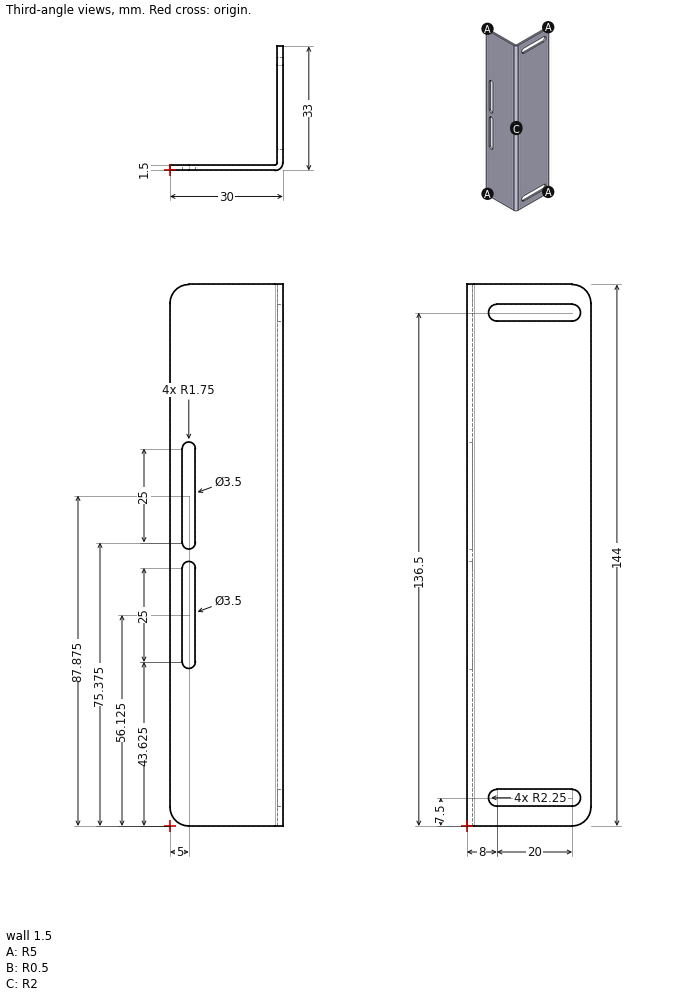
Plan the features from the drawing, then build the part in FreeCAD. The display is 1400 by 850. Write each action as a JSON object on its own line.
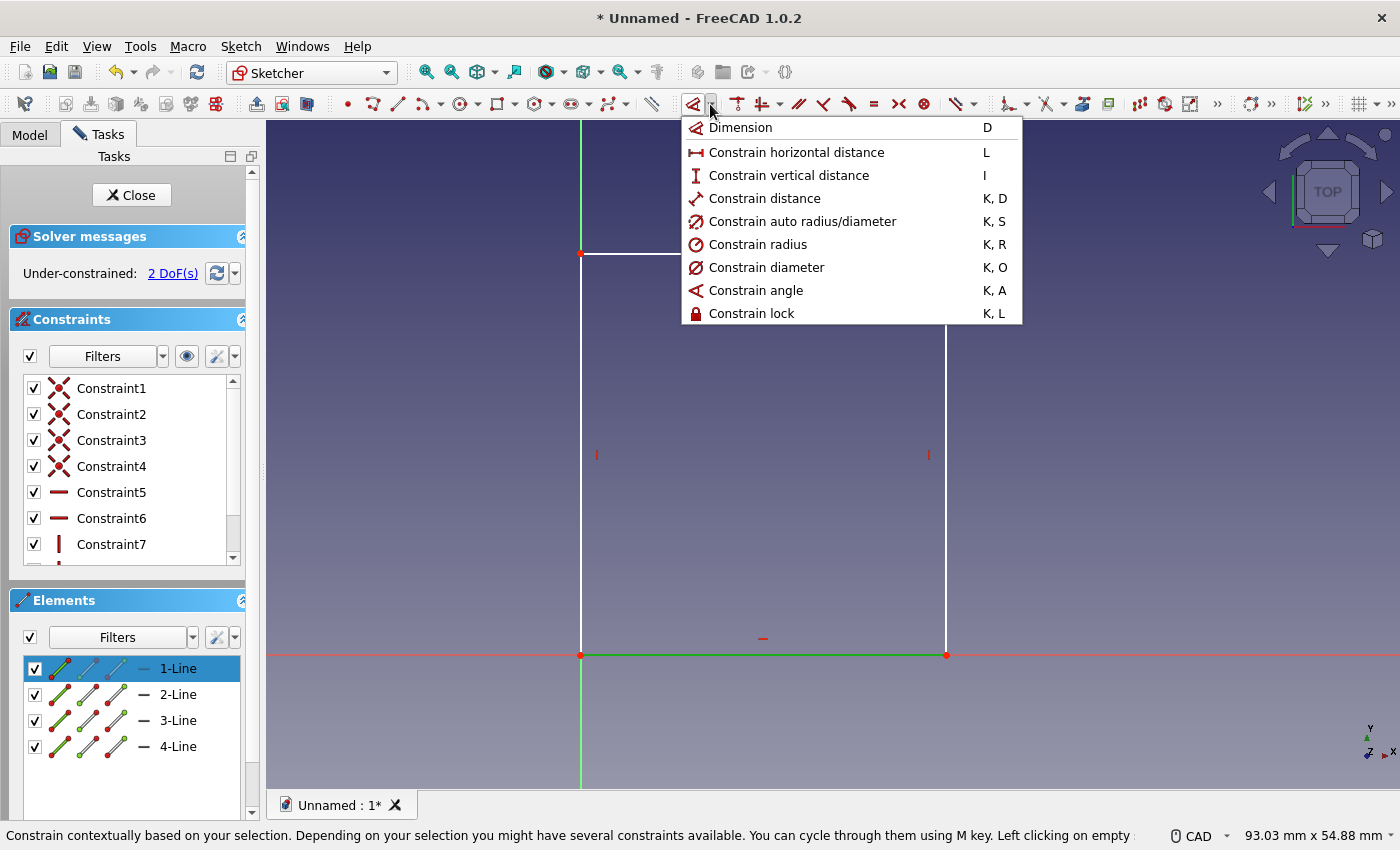
{"action": "left_click", "coordinate": [852, 152]}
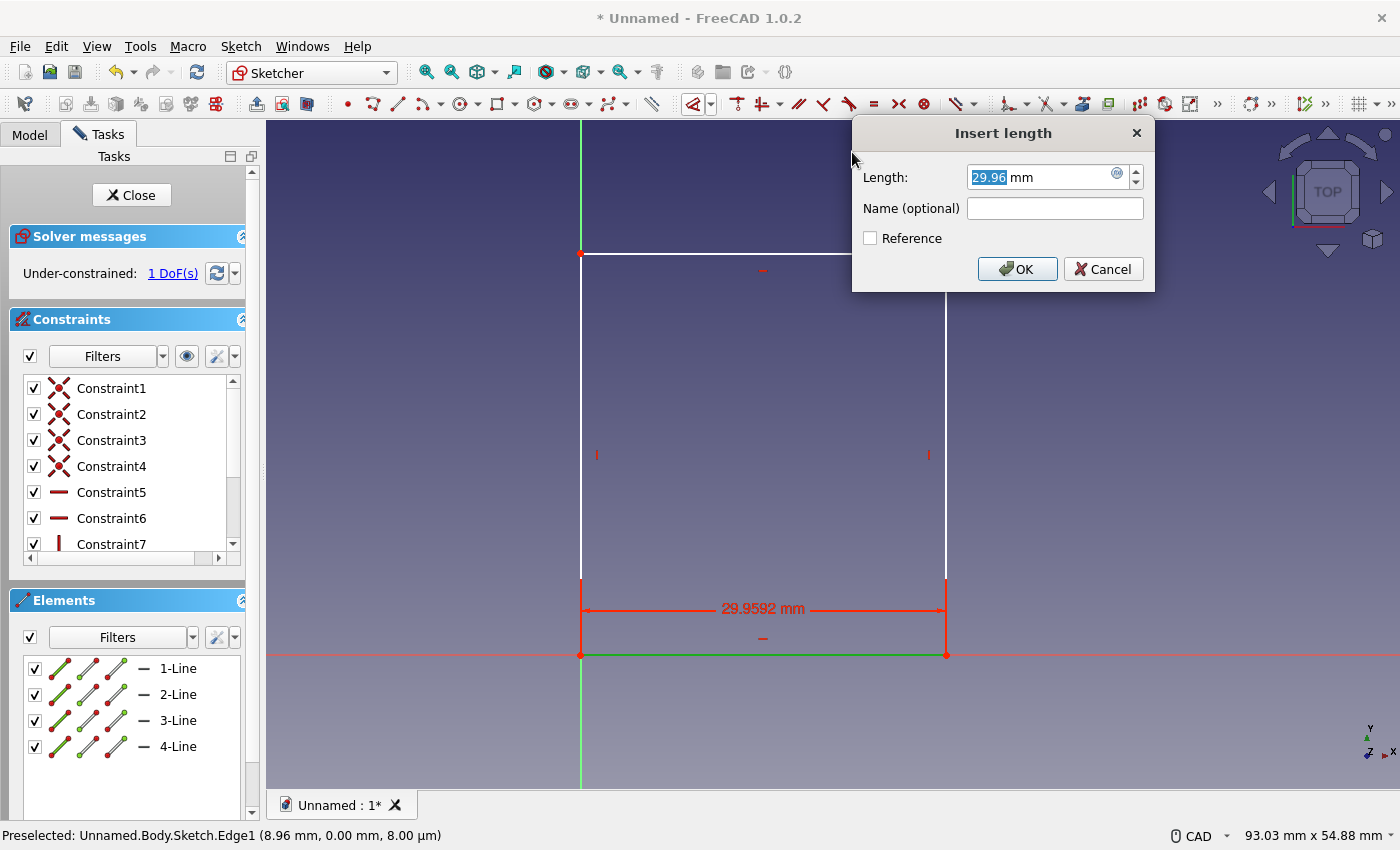
{"action": "type", "text": "30"}
{"action": "key", "text": "Return"}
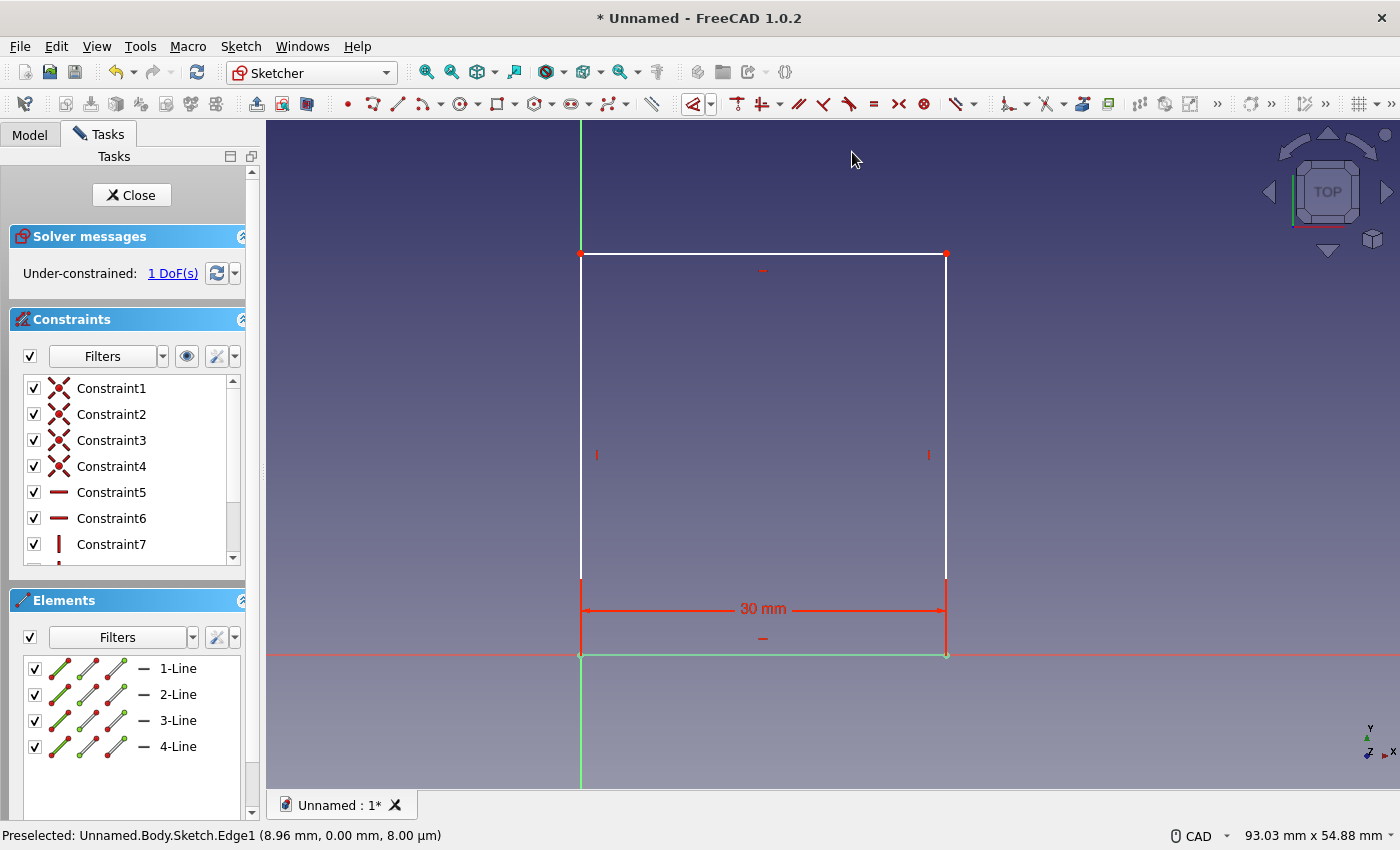
{"action": "left_click", "coordinate": [946, 535]}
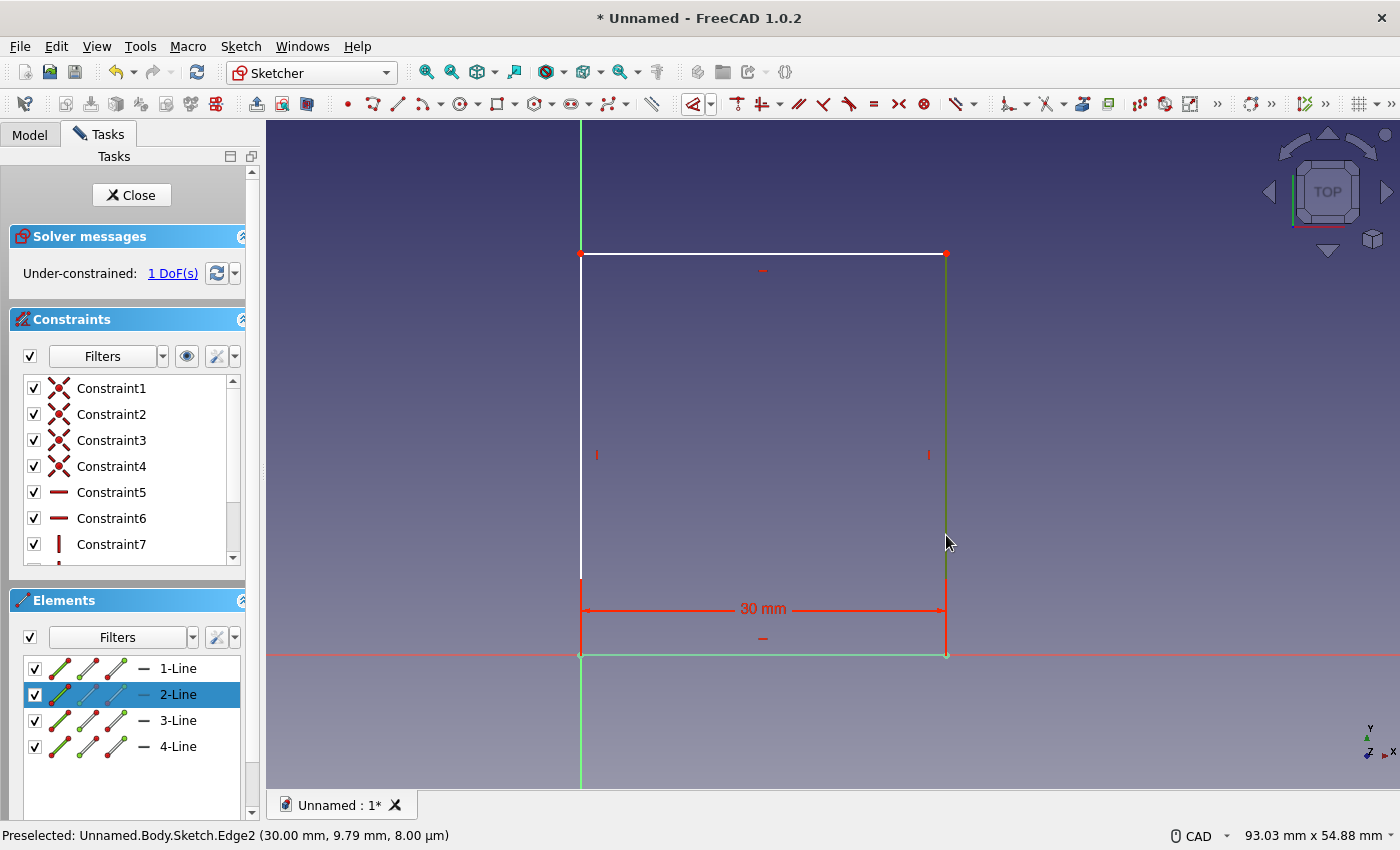
{"action": "key", "text": "i"}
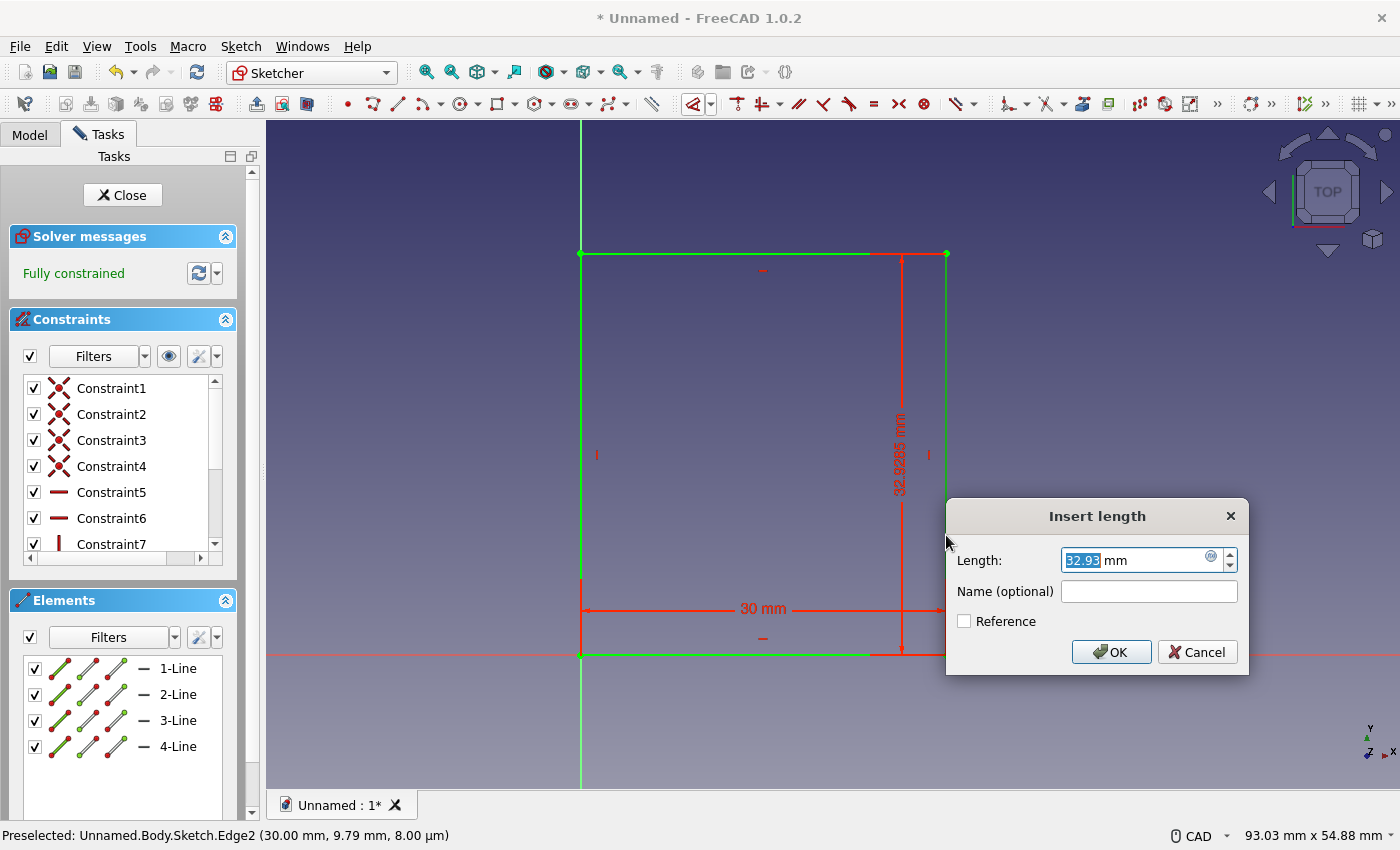
{"action": "type", "text": "33"}
{"action": "key", "text": "Return"}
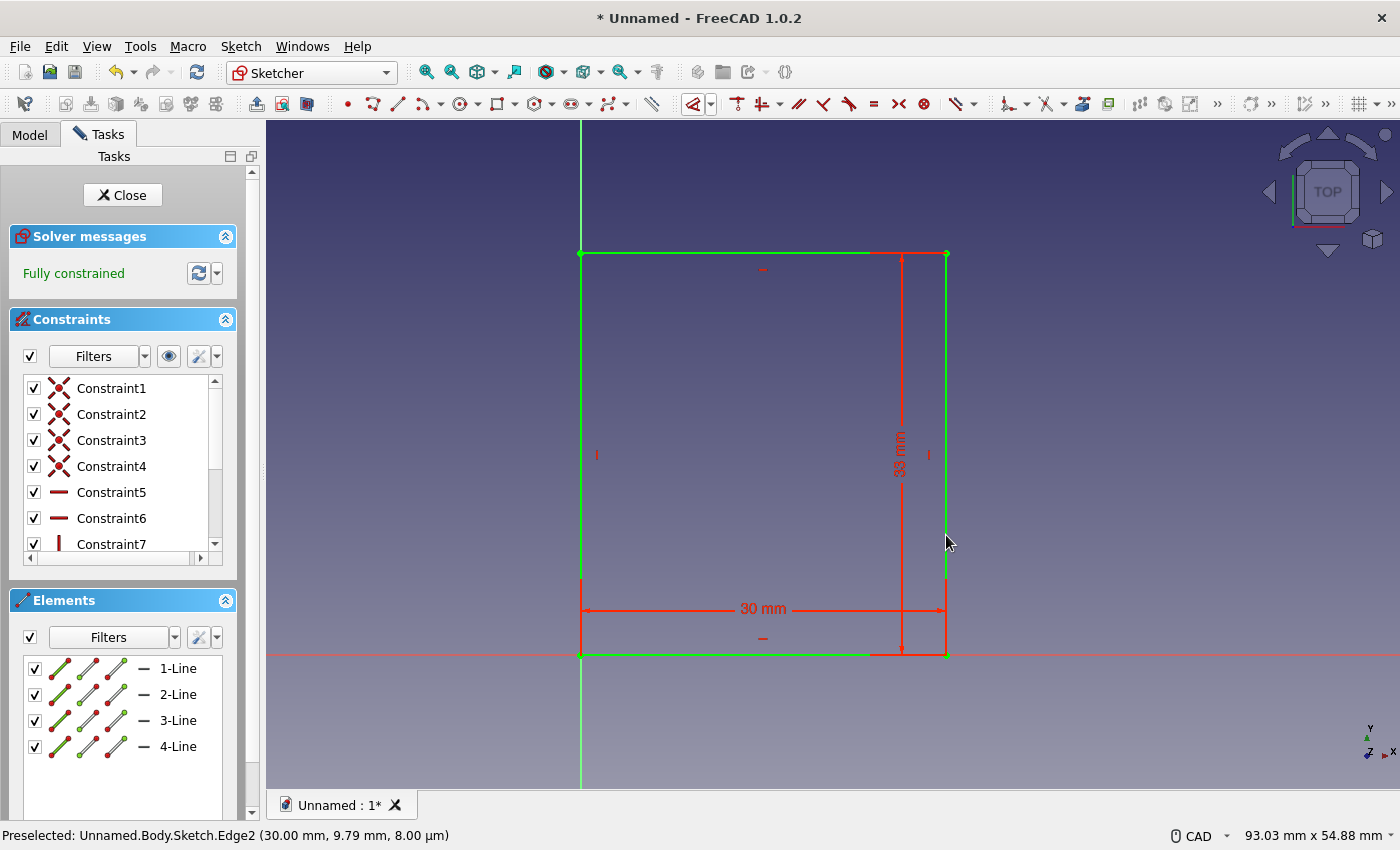
{"action": "left_click", "coordinate": [123, 195]}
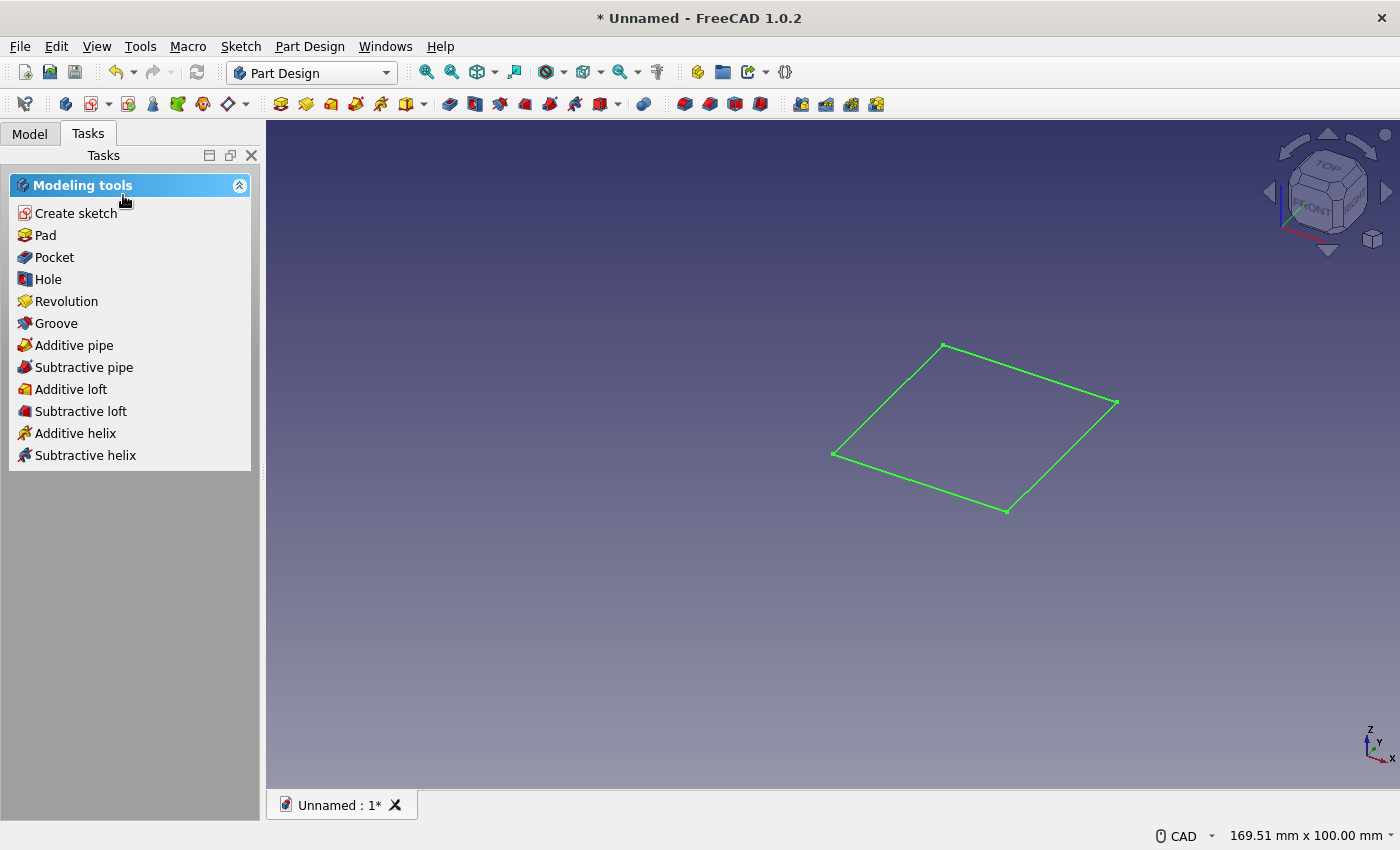
{"action": "left_click", "coordinate": [281, 104]}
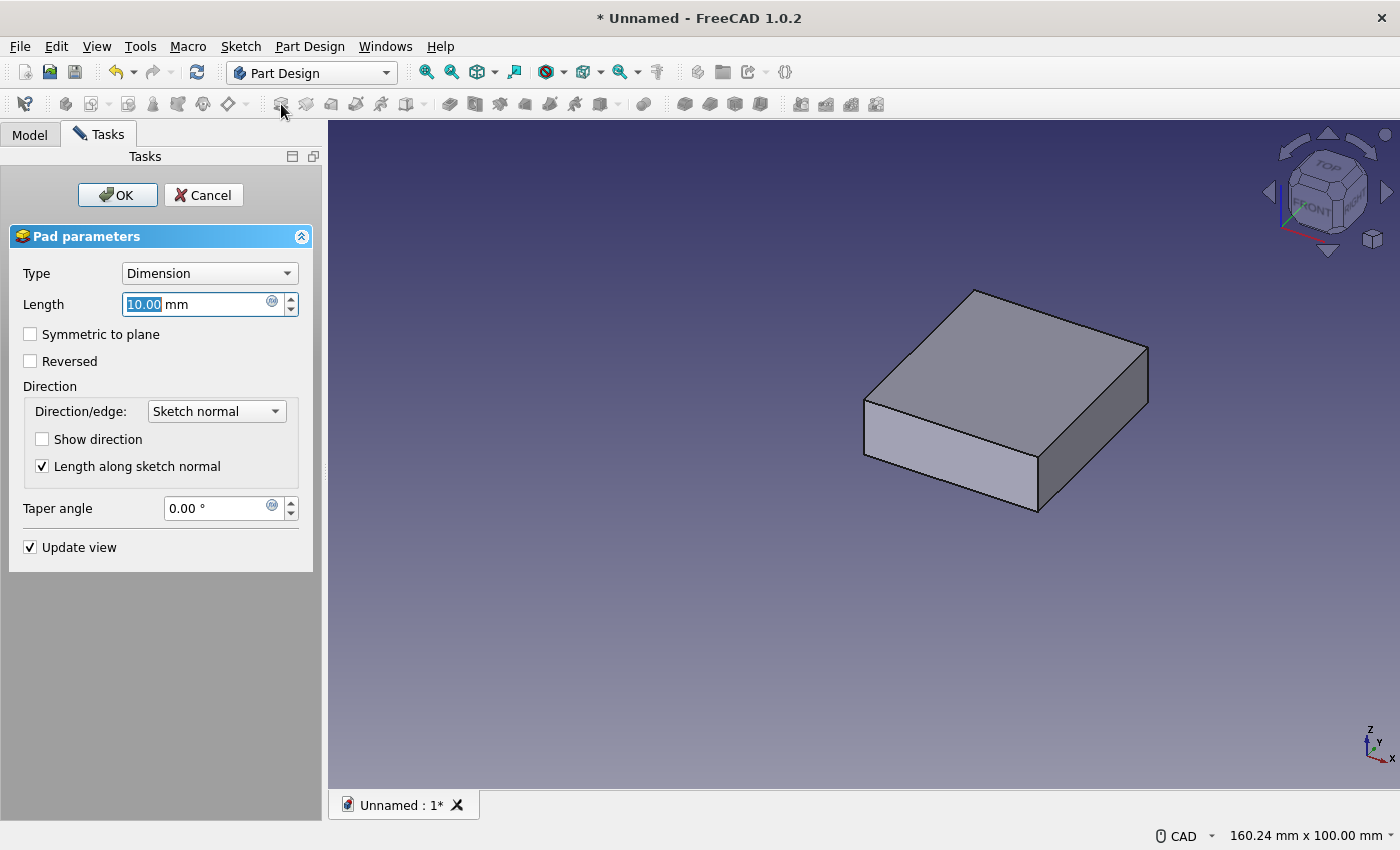
{"action": "type", "text": "144"}
{"action": "key", "text": "Tab"}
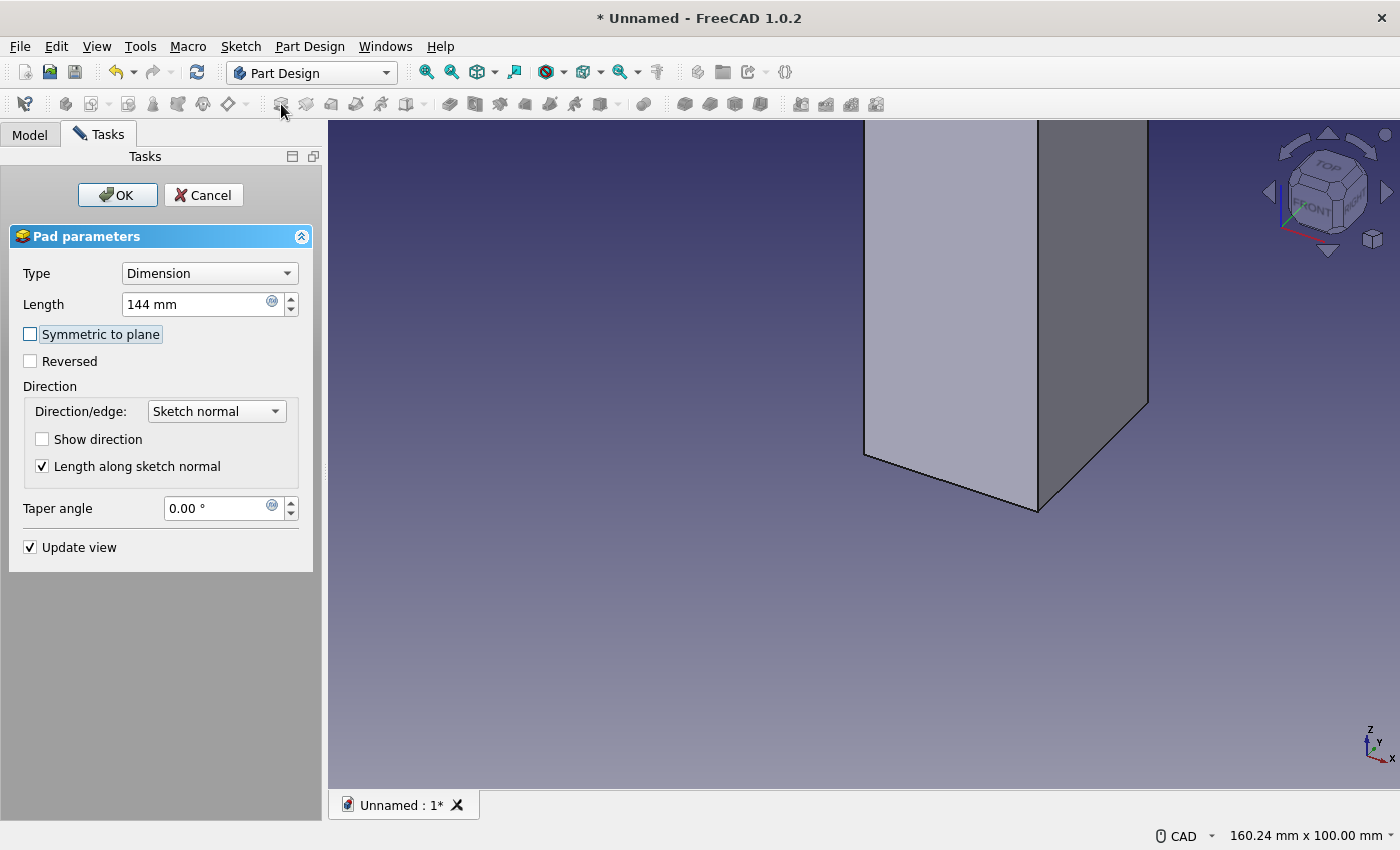
{"action": "left_click", "coordinate": [118, 195]}